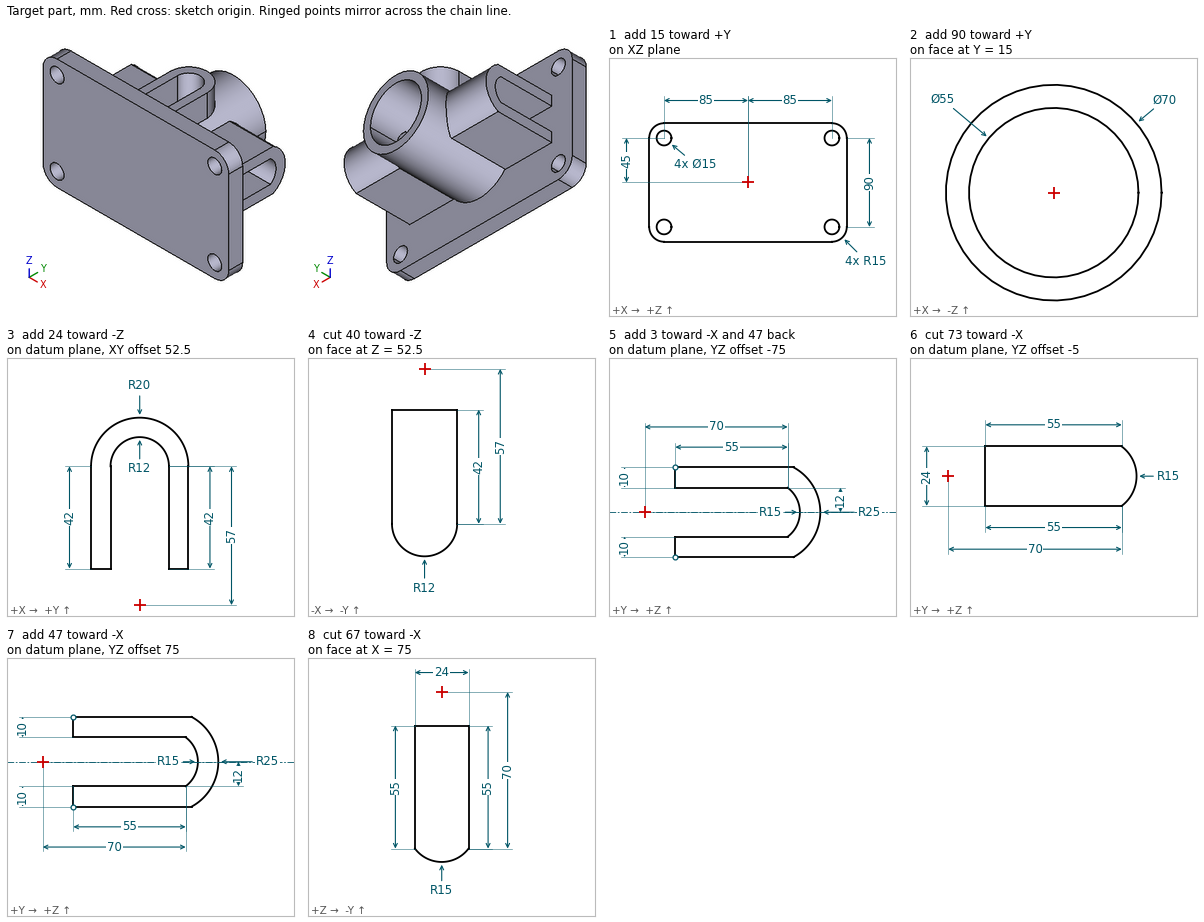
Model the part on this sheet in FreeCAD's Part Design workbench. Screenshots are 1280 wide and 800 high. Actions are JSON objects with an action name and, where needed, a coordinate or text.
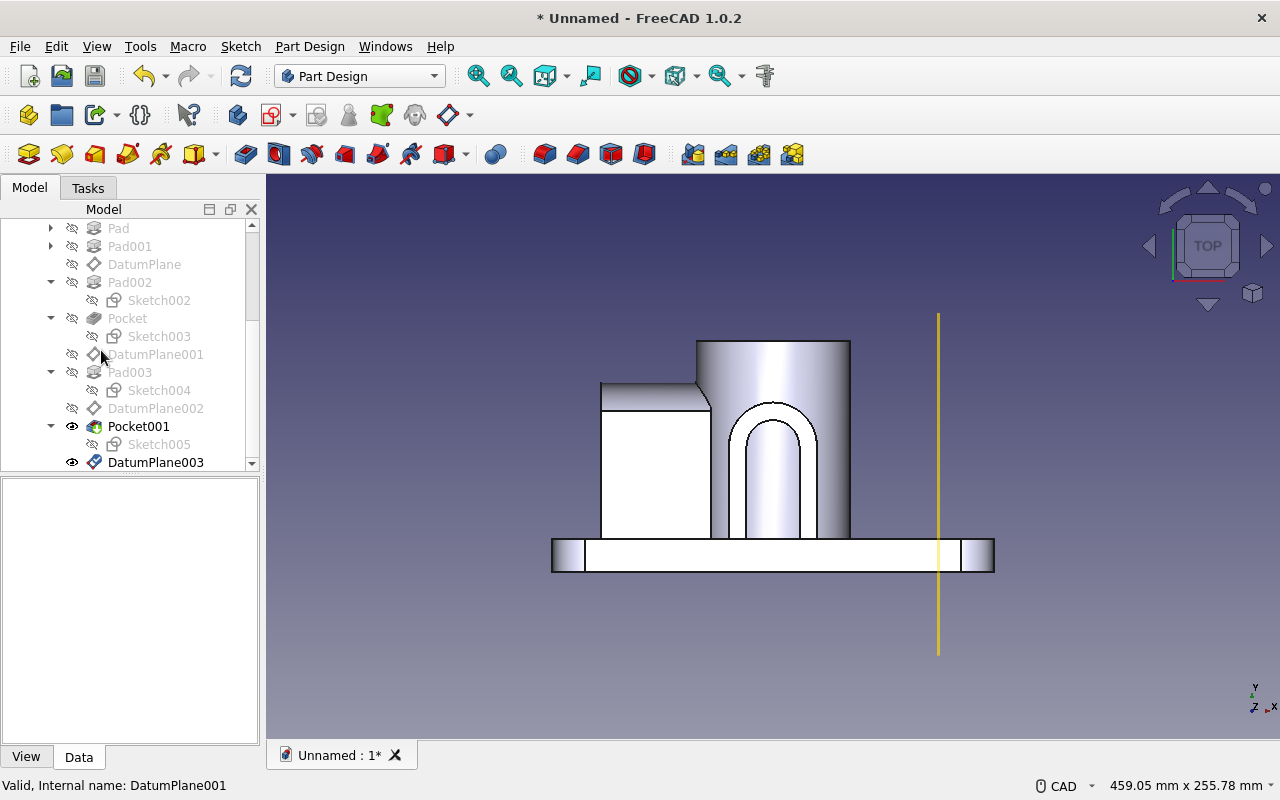
{"action": "left_click", "coordinate": [117, 462]}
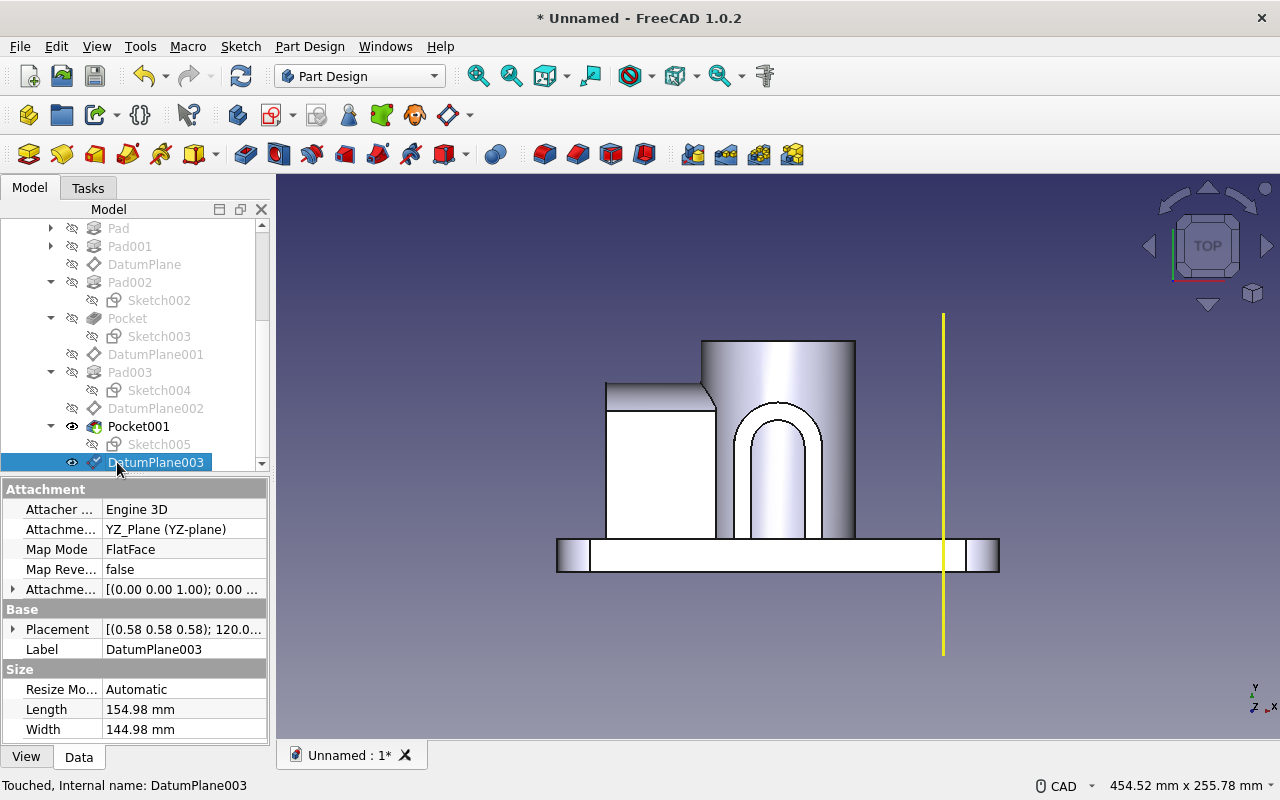
{"action": "left_click", "coordinate": [270, 116]}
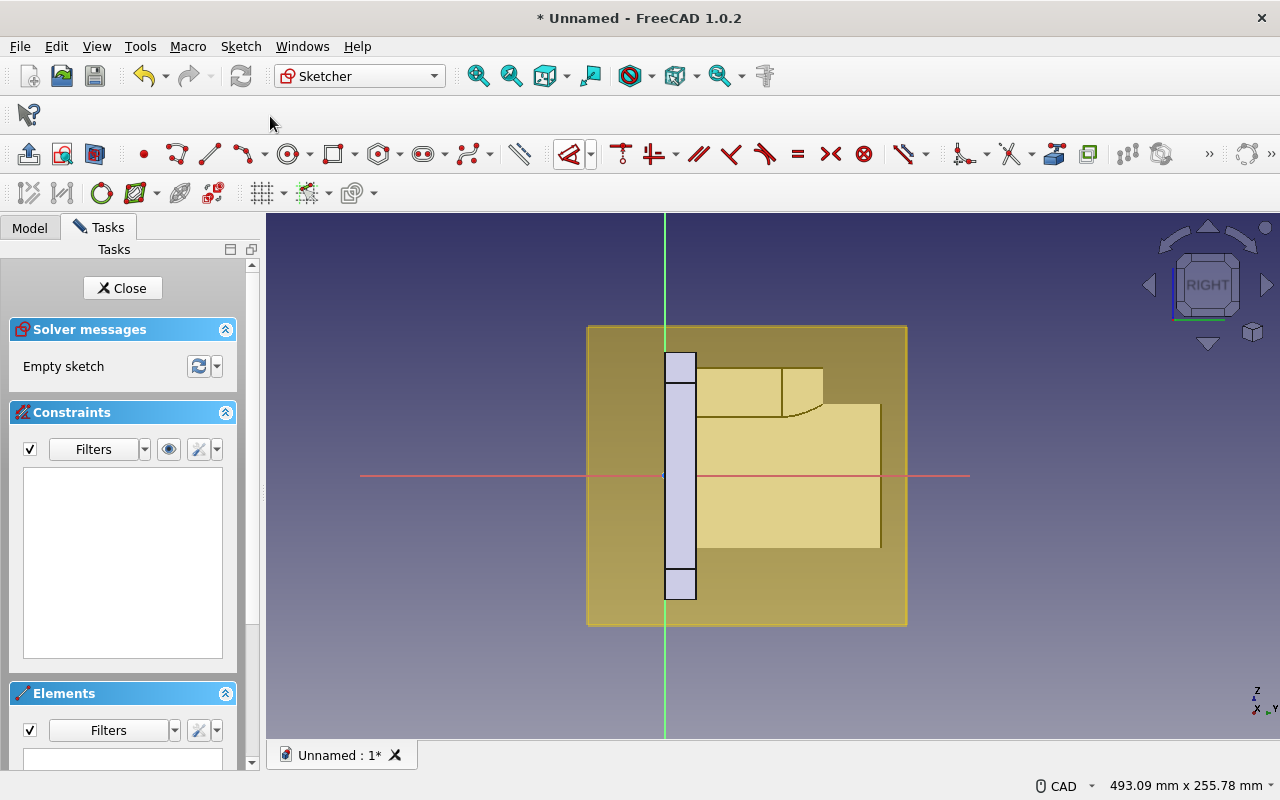
{"action": "left_click", "coordinate": [95, 154]}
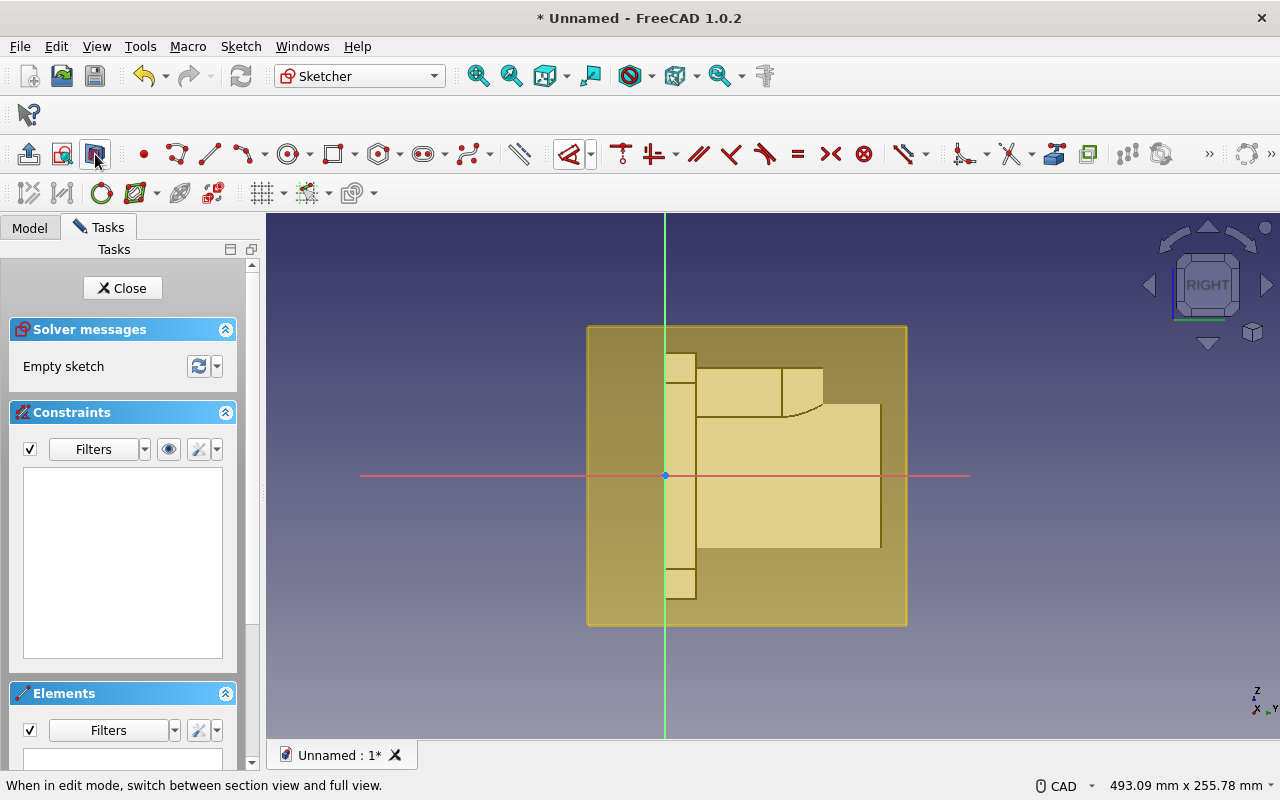
{"action": "scroll", "coordinate": [775, 476], "scroll_direction": "up", "scroll_amount": 6}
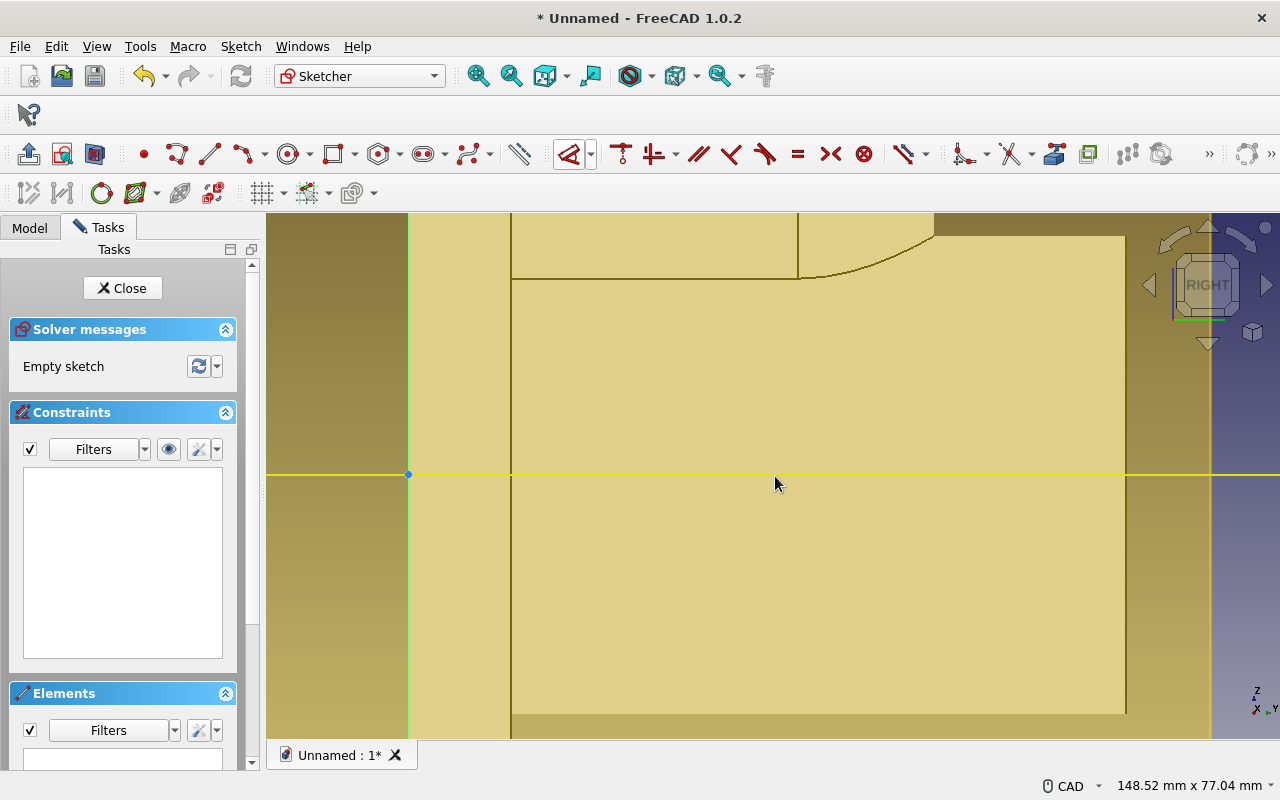
{"action": "left_click", "coordinate": [177, 154]}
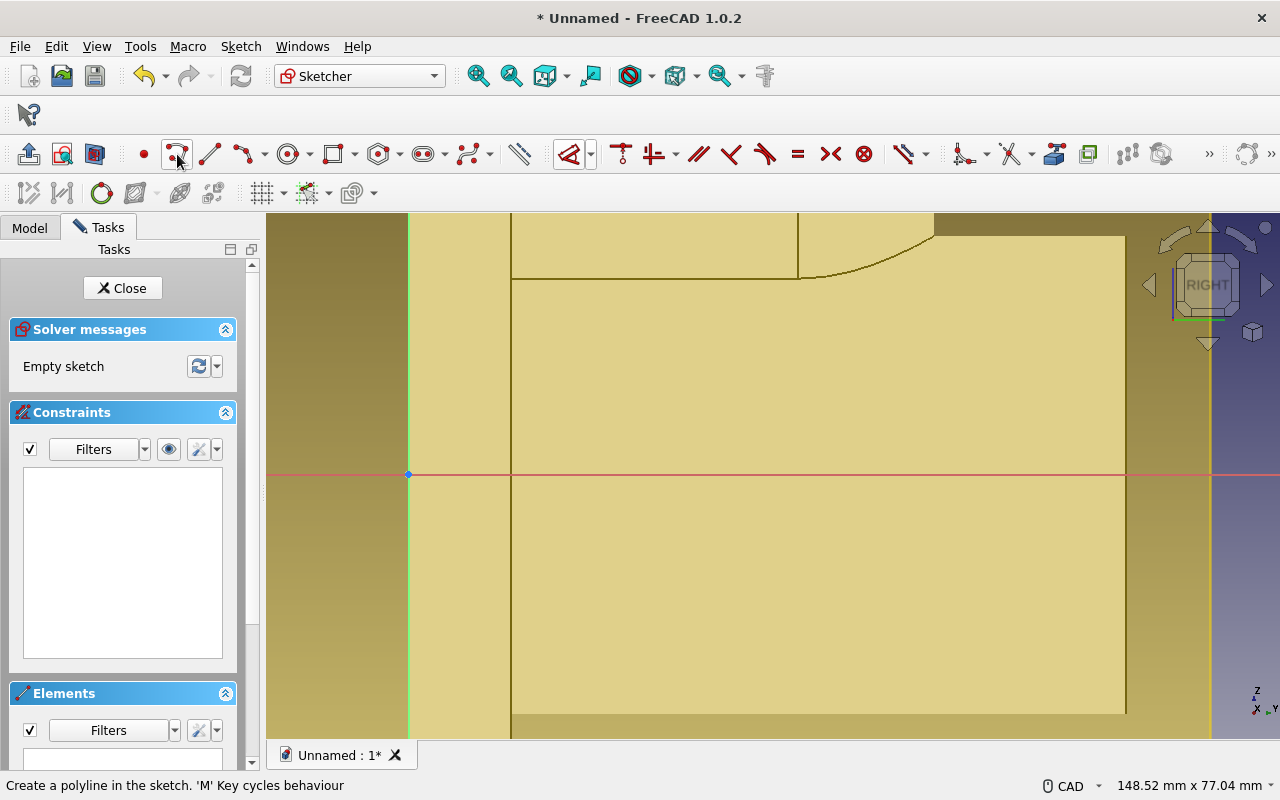
{"action": "left_click", "coordinate": [887, 557]}
{"action": "left_click", "coordinate": [511, 557]}
{"action": "left_click", "coordinate": [511, 625]}
{"action": "left_click", "coordinate": [906, 625]}
{"action": "right_click", "coordinate": [906, 625]}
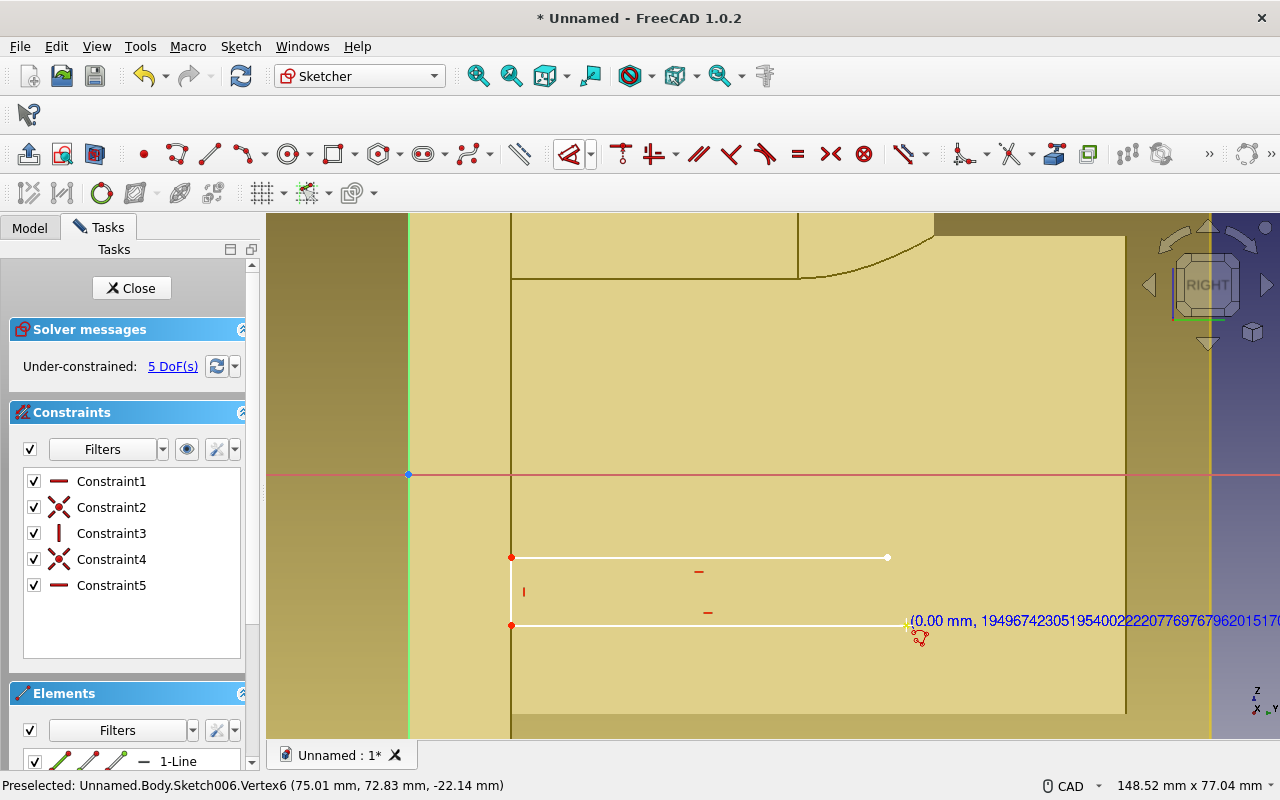
{"action": "left_click", "coordinate": [906, 325]}
{"action": "left_click", "coordinate": [511, 325]}
{"action": "left_click", "coordinate": [511, 393]}
{"action": "left_click", "coordinate": [887, 393]}
{"action": "right_click", "coordinate": [887, 393]}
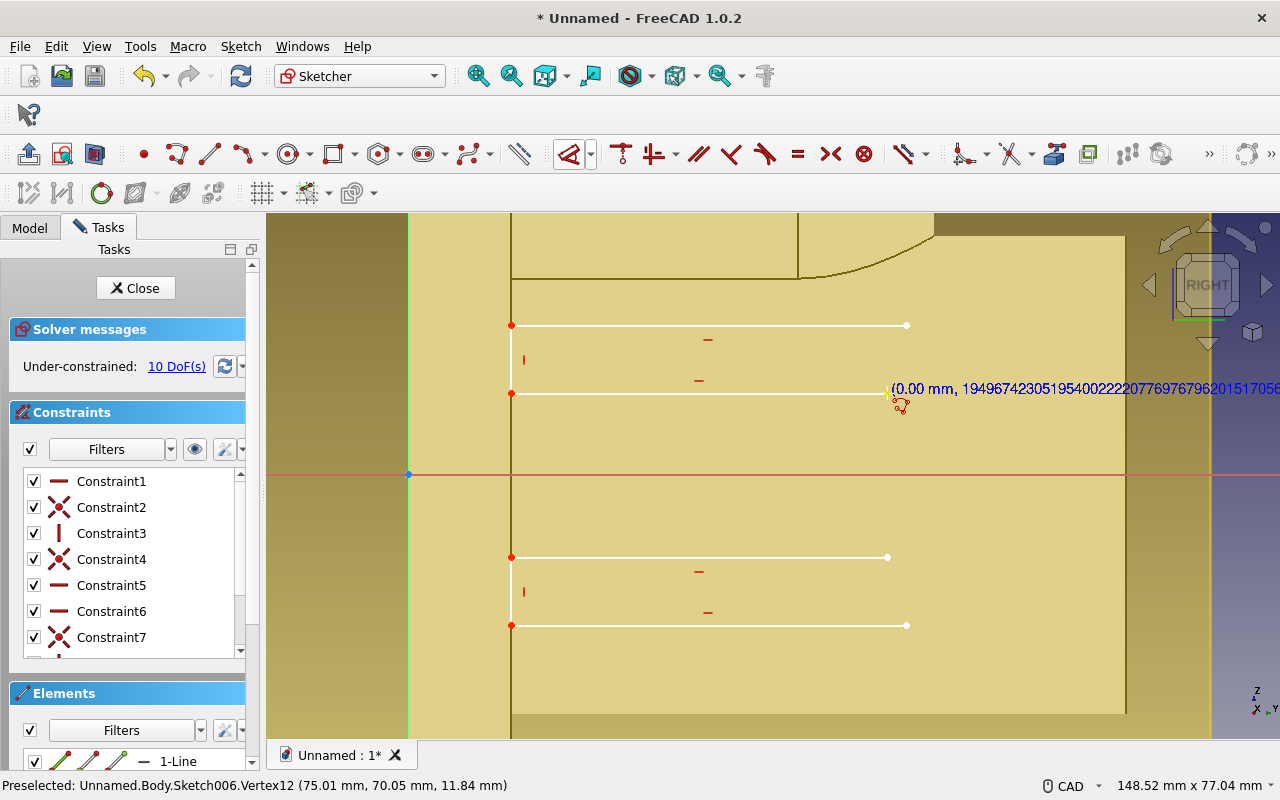
{"action": "left_click", "coordinate": [242, 154]}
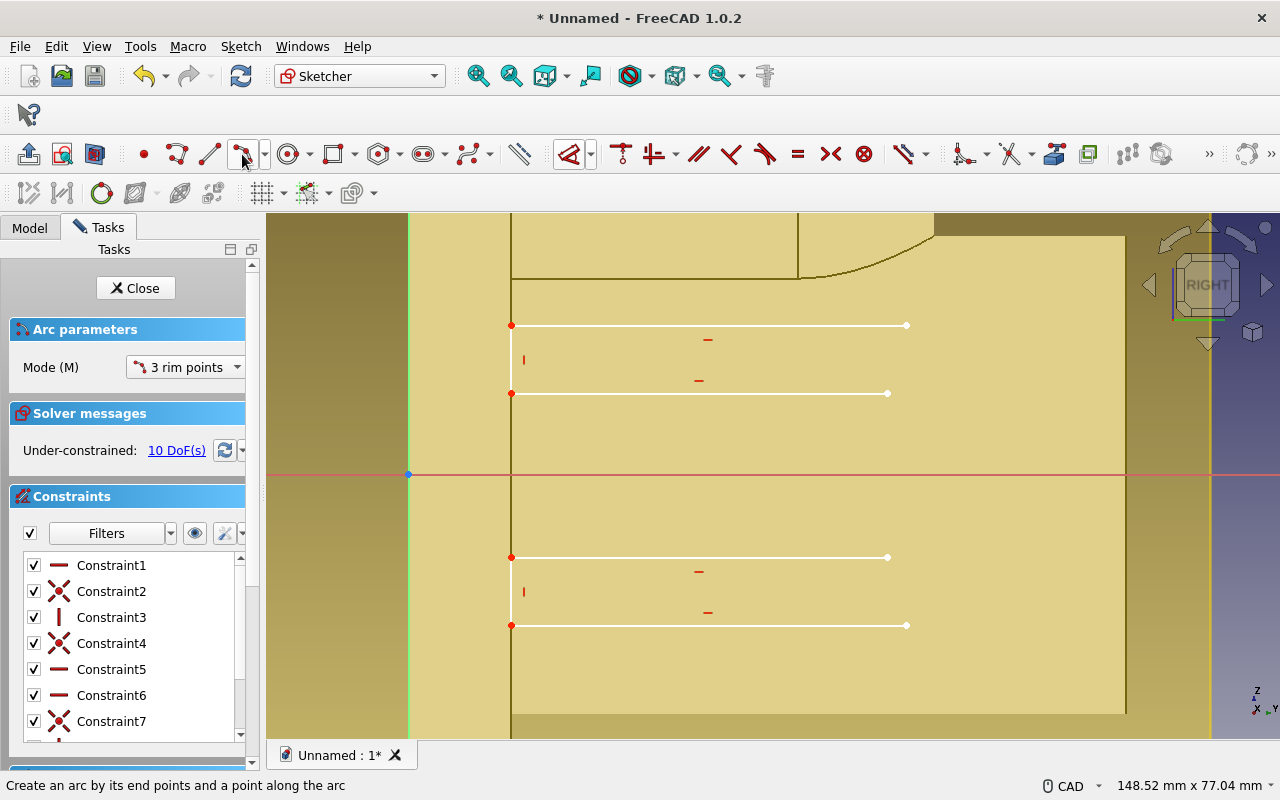
{"action": "left_click", "coordinate": [906, 626]}
{"action": "left_click", "coordinate": [906, 326]}
{"action": "left_click", "coordinate": [992, 511]}